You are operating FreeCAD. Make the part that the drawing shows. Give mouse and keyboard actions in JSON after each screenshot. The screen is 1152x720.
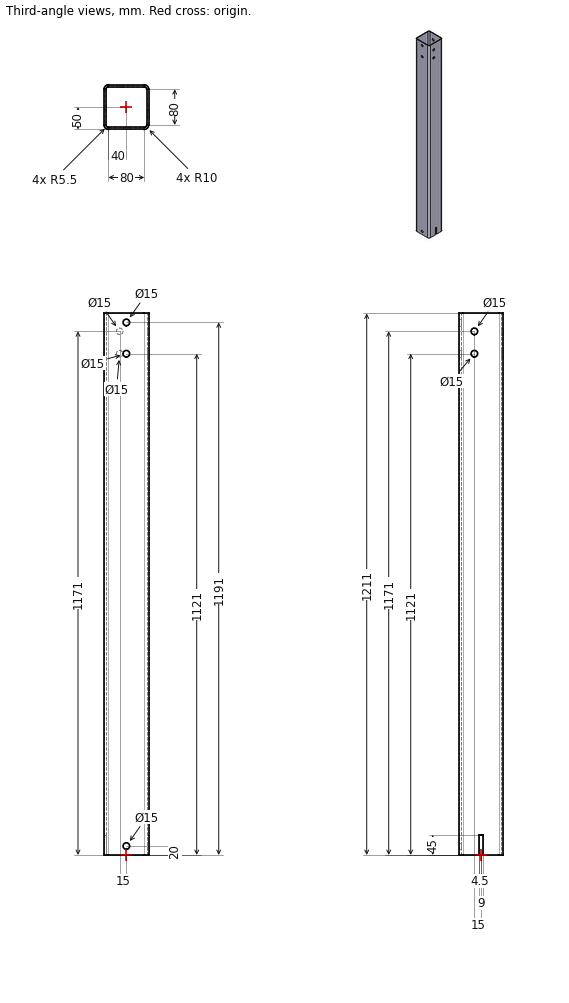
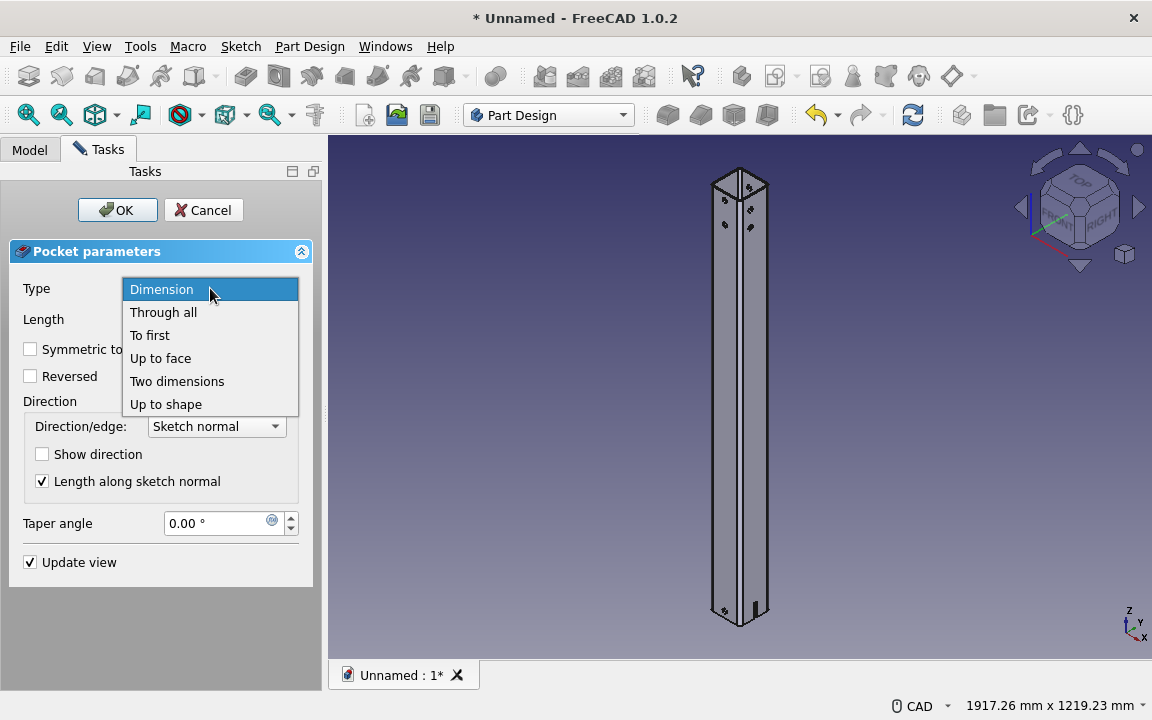
{"action": "left_click", "coordinate": [208, 312]}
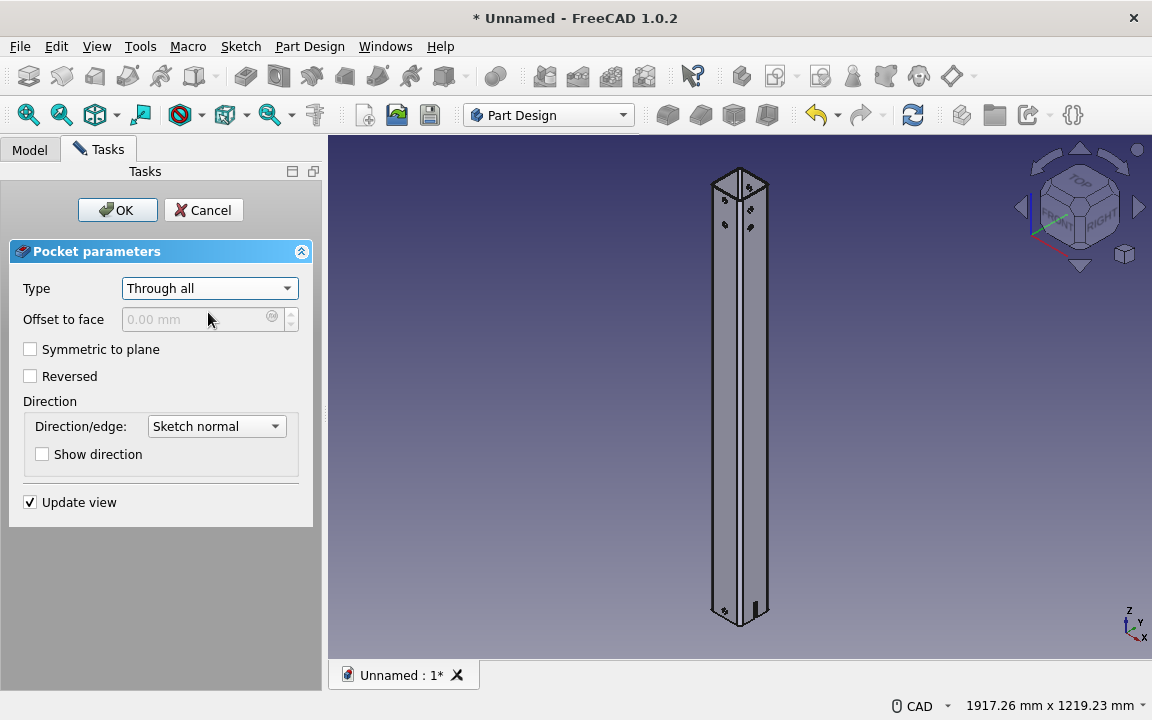
{"action": "left_click", "coordinate": [118, 210]}